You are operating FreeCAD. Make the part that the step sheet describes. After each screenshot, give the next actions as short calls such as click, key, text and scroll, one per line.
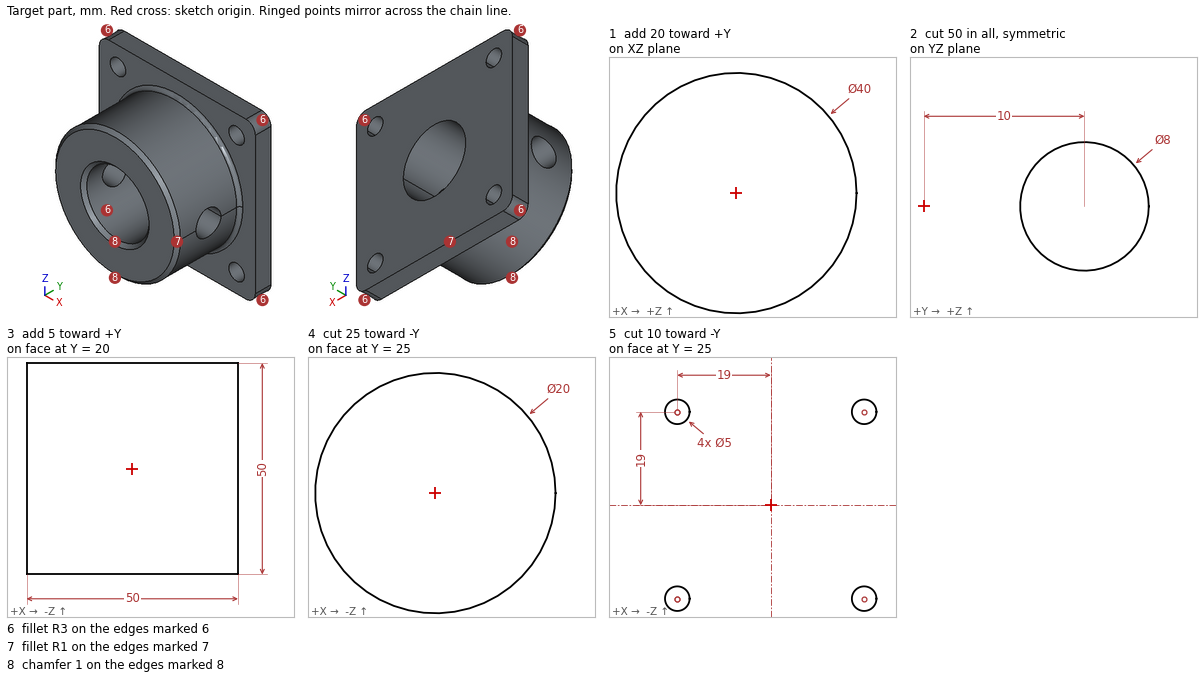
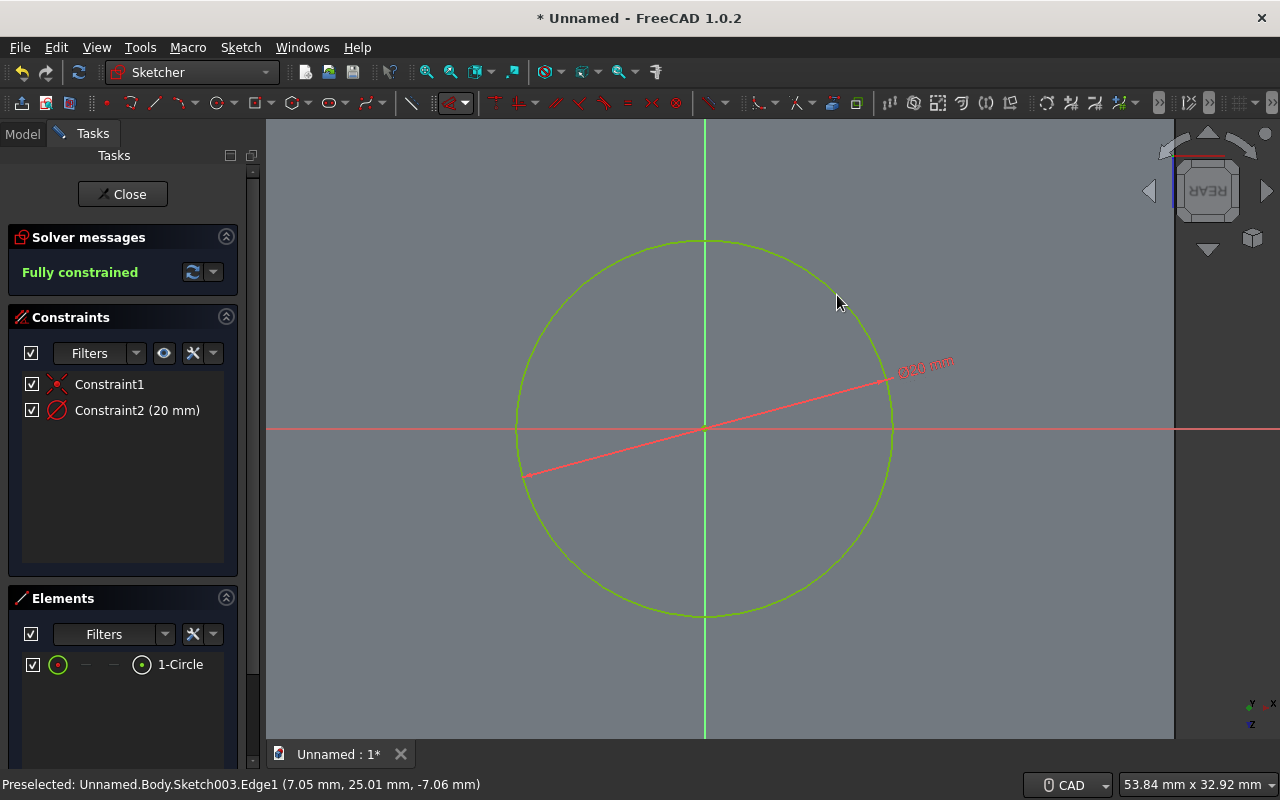
click(123, 194)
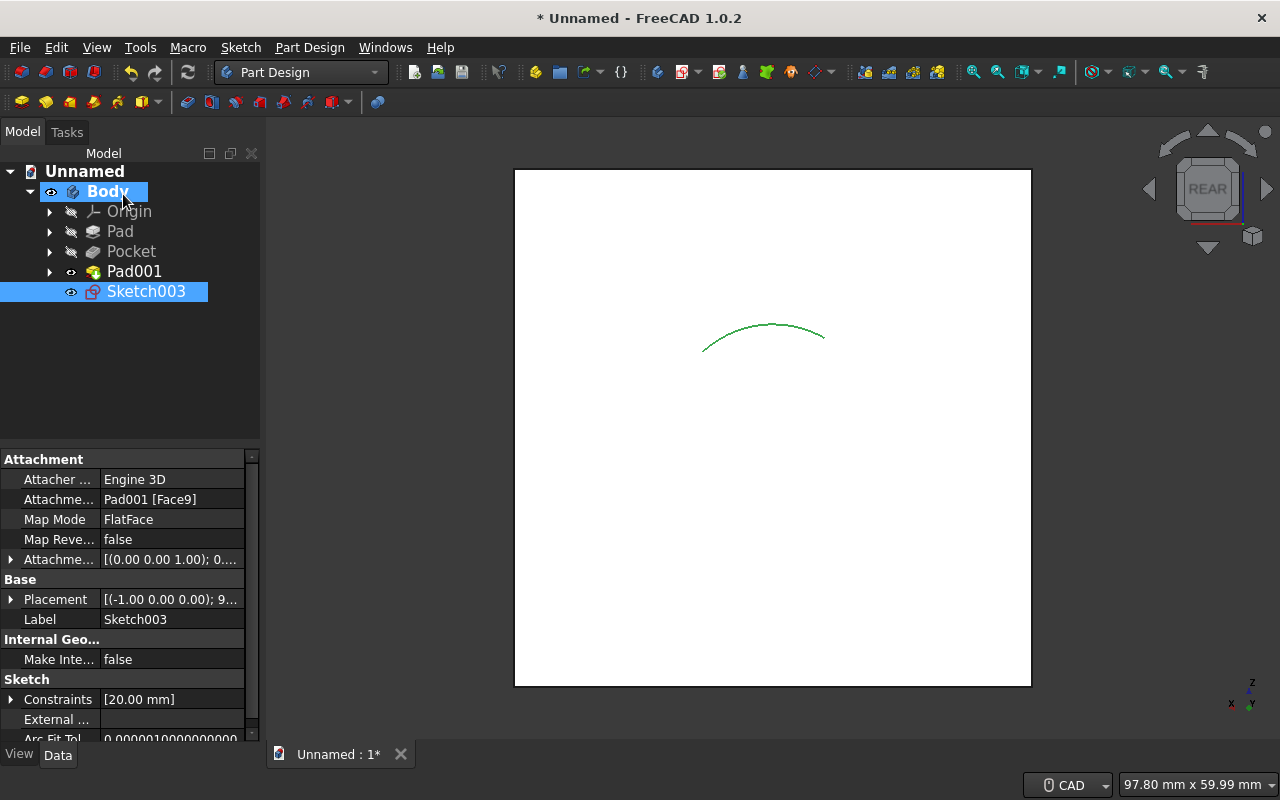
click(188, 102)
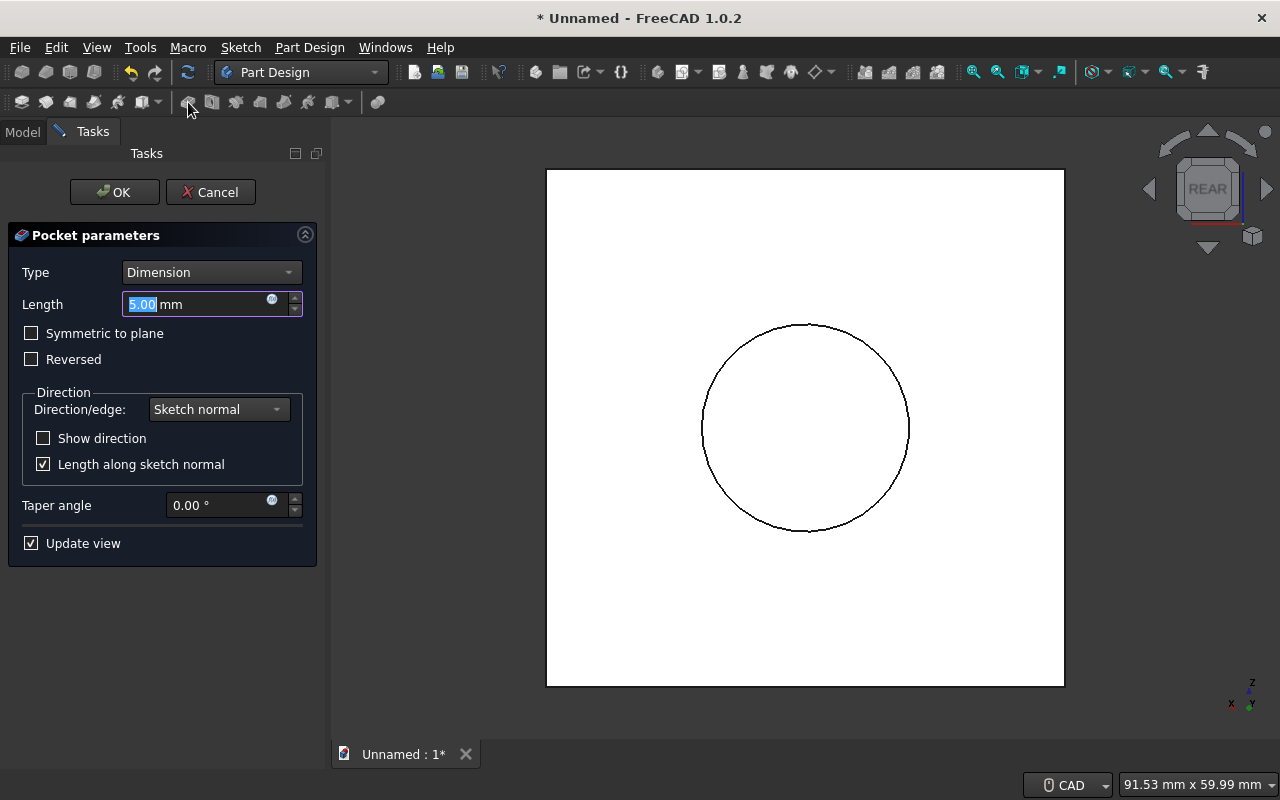
text(25)
key(Tab)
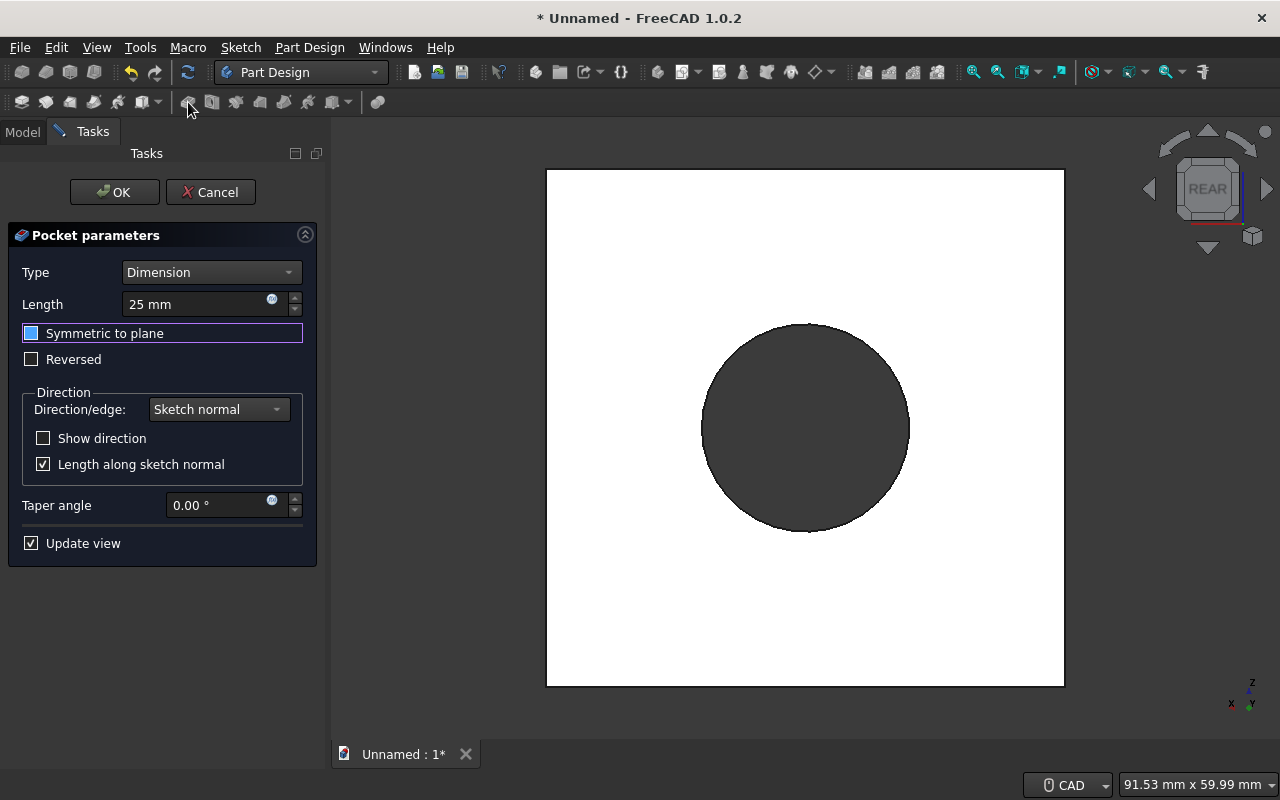
click(115, 192)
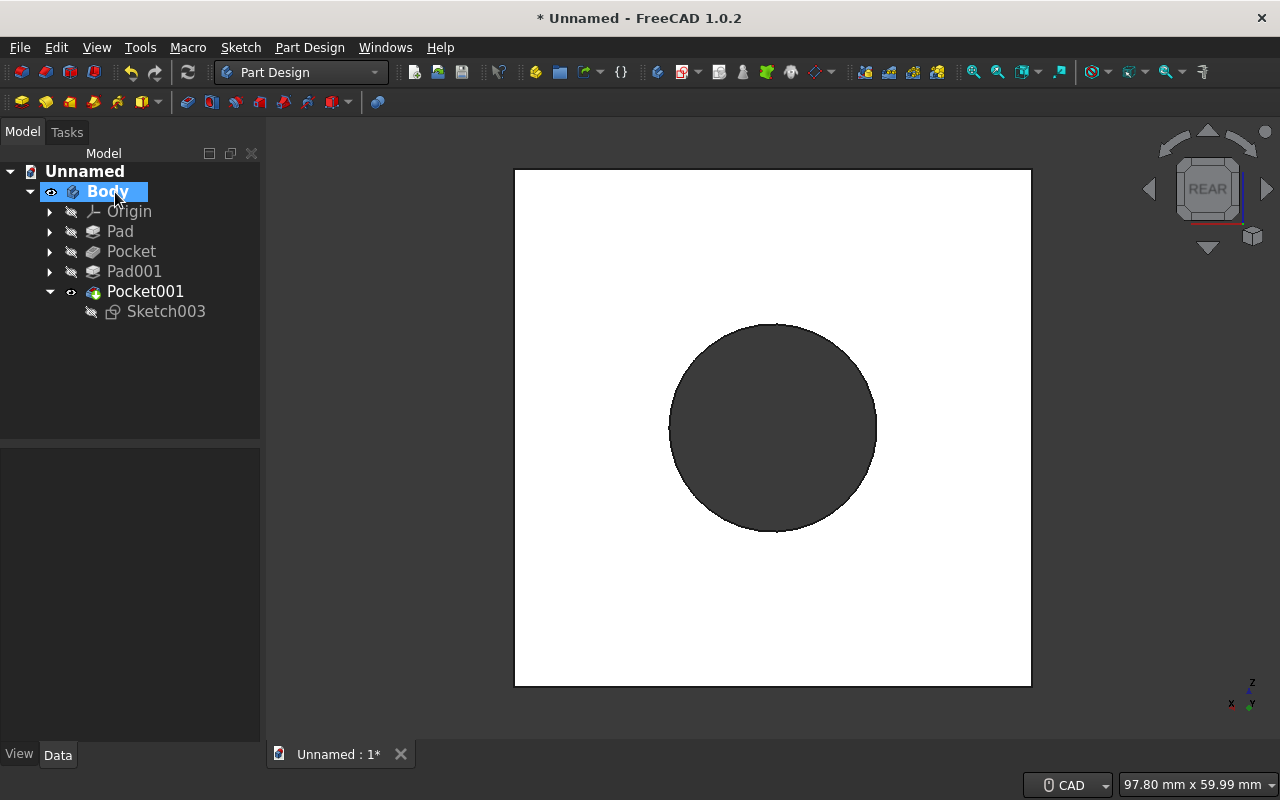
click(921, 575)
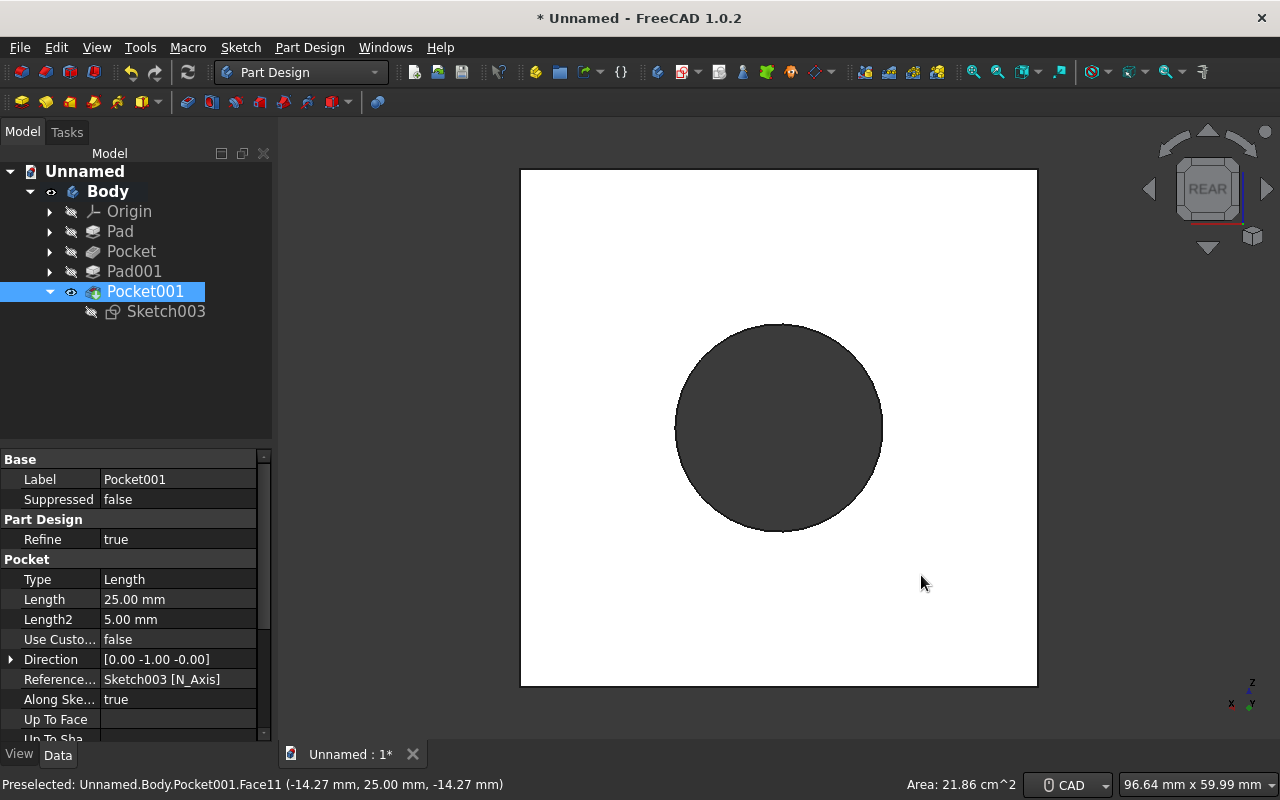
click(682, 72)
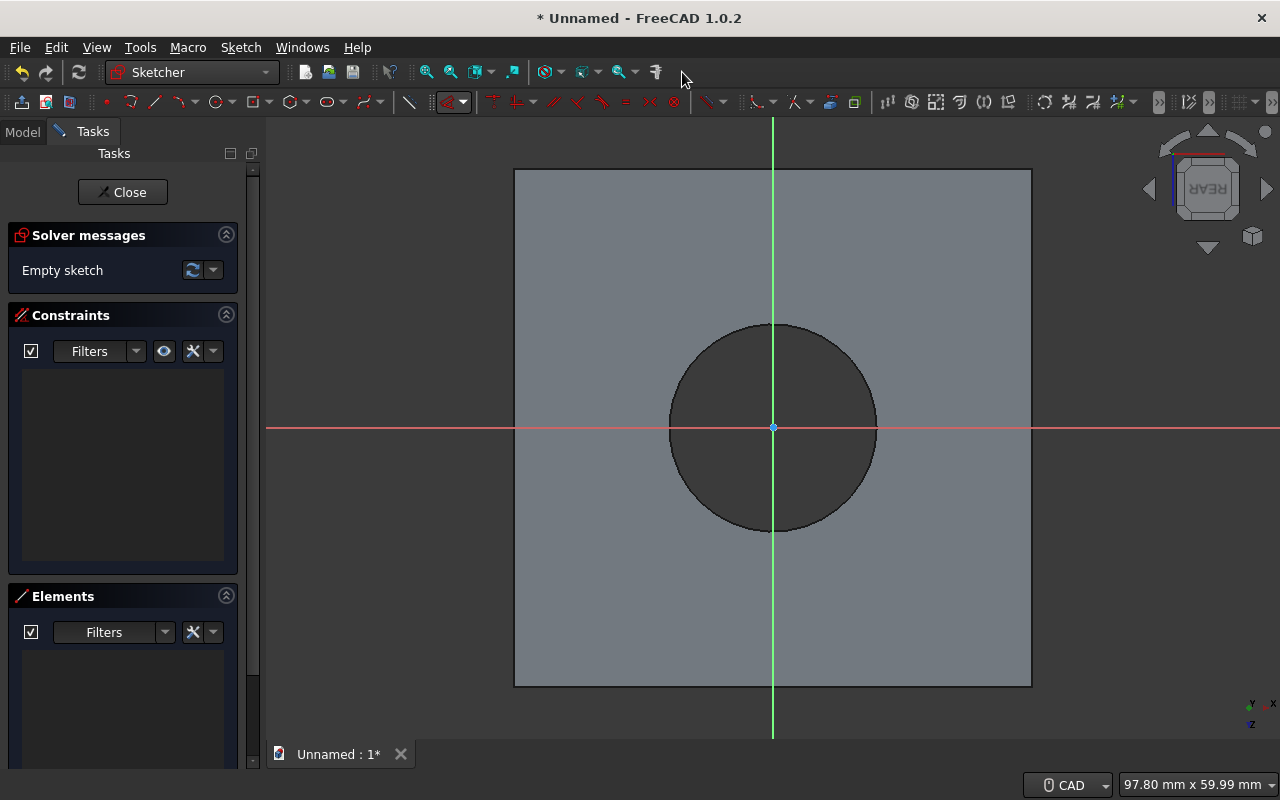
click(216, 102)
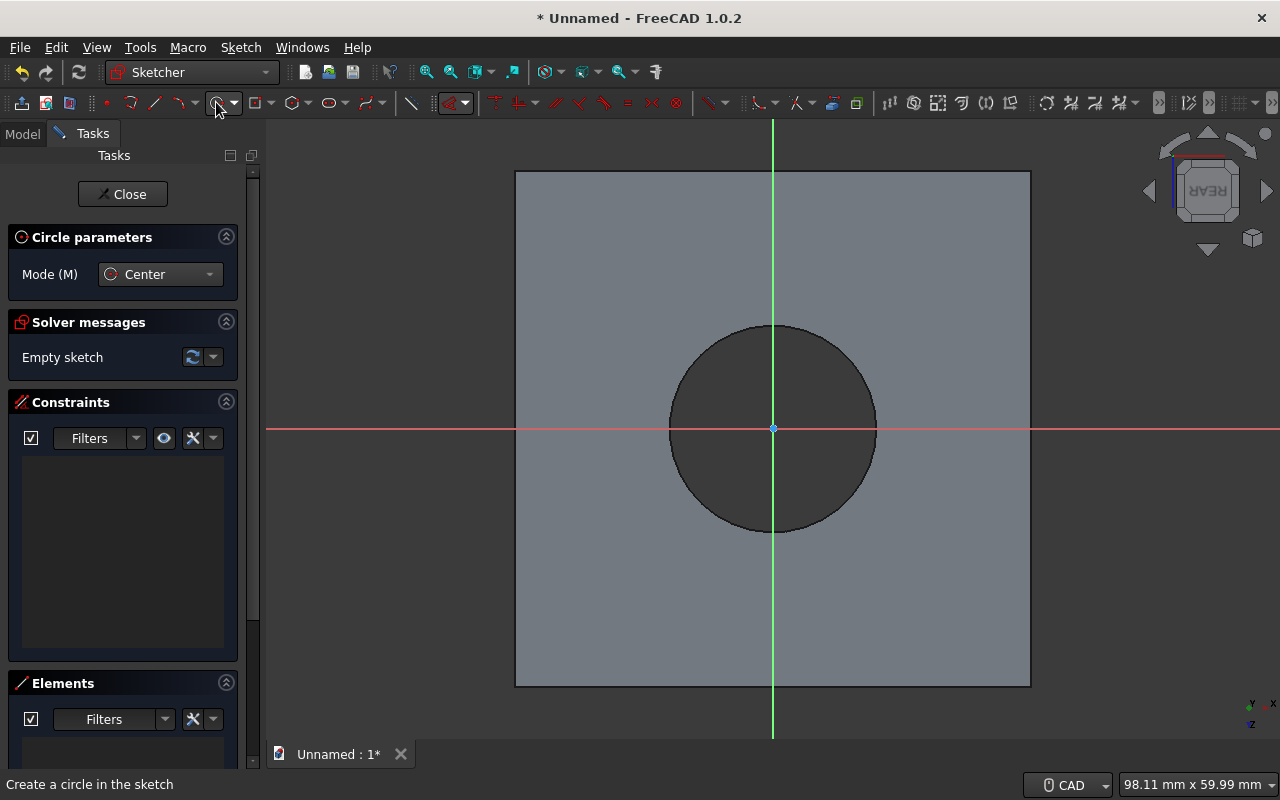
click(577, 233)
click(595, 214)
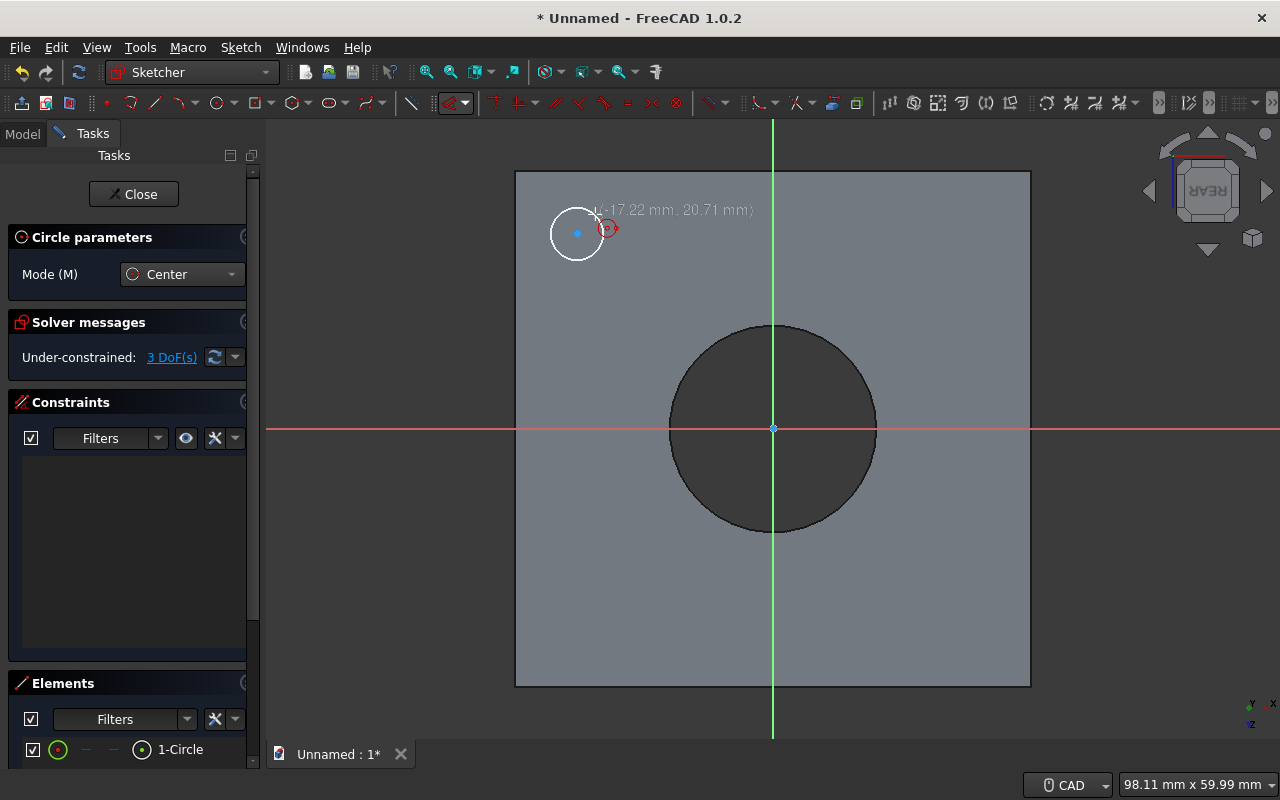
click(577, 625)
click(595, 607)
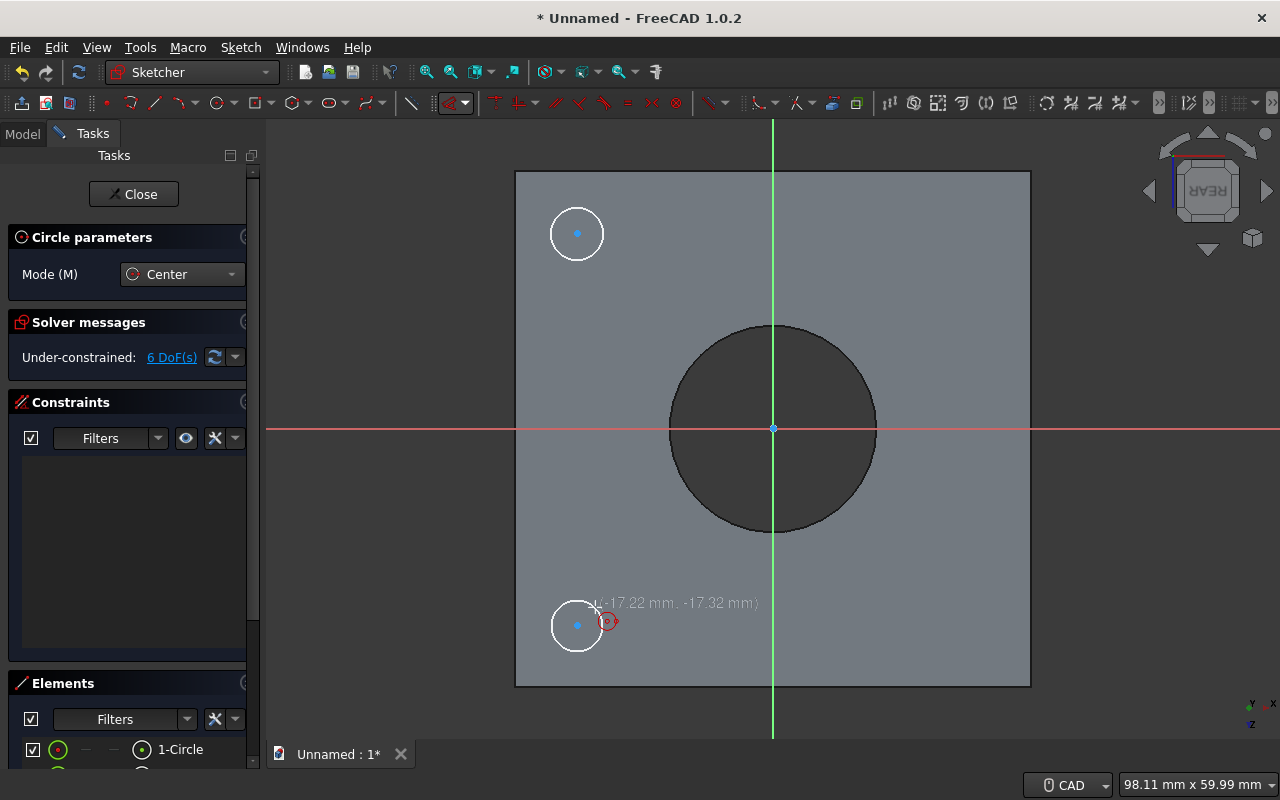
click(969, 625)
click(988, 607)